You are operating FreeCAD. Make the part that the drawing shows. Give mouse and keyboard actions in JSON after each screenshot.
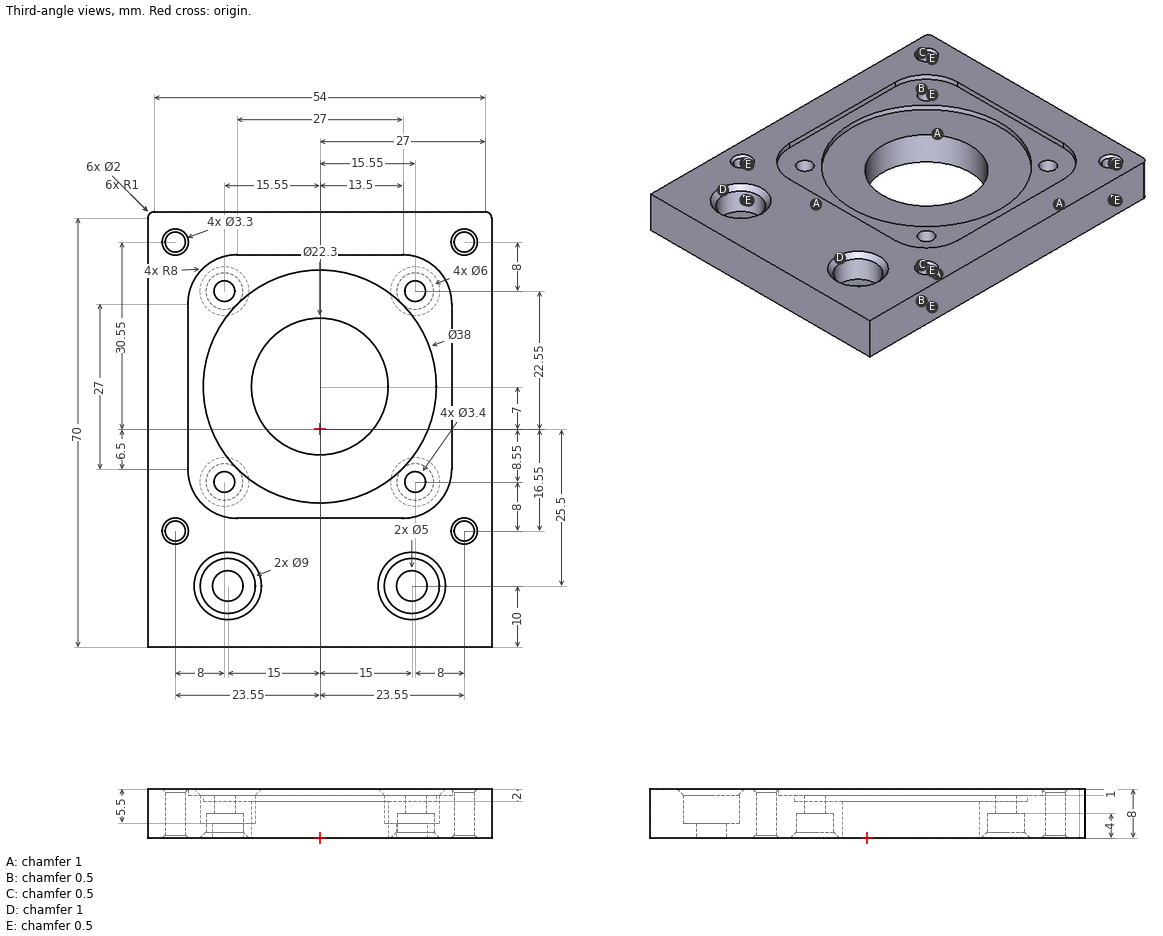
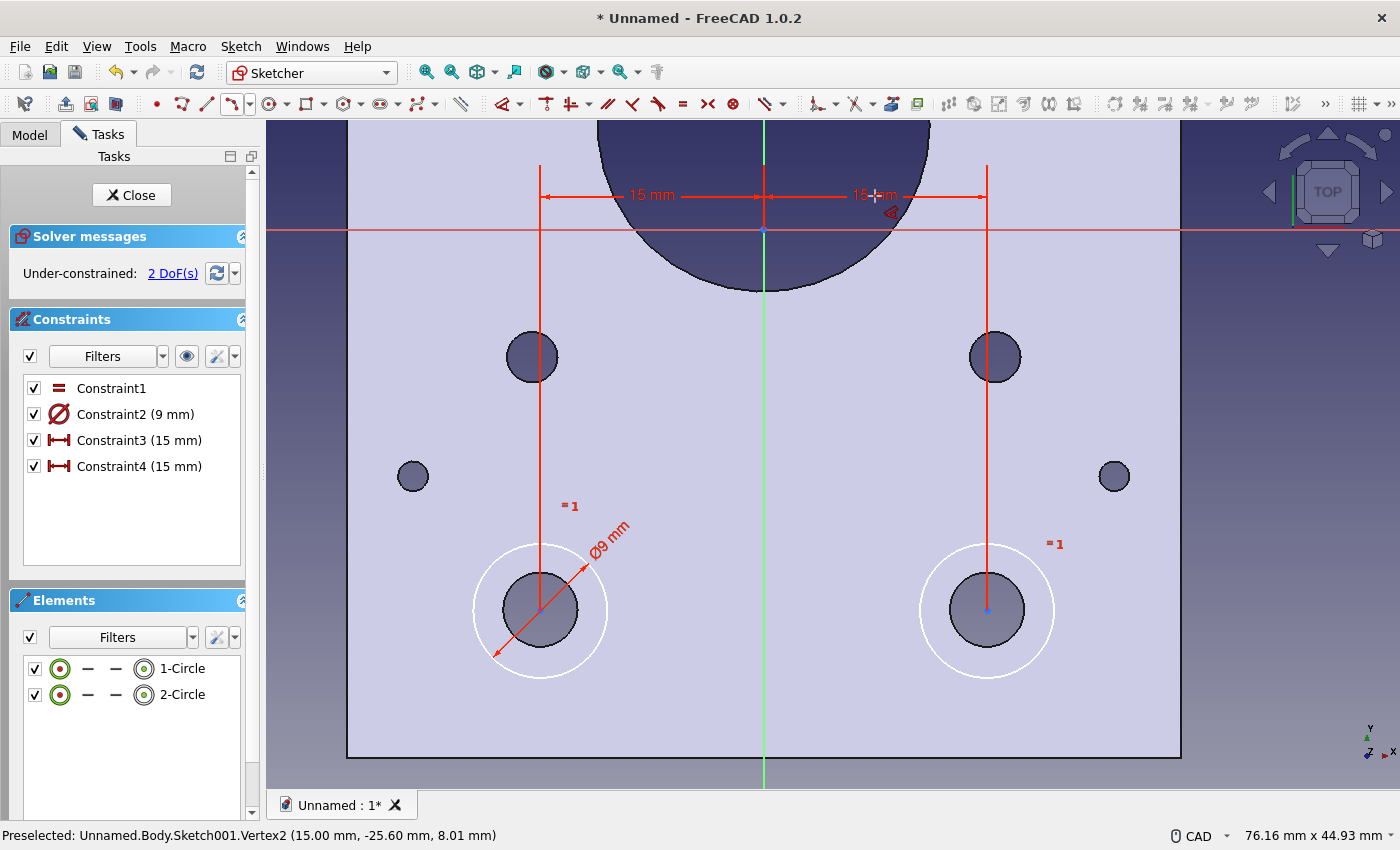
{"action": "left_click", "coordinate": [540, 611]}
{"action": "left_click", "coordinate": [506, 420]}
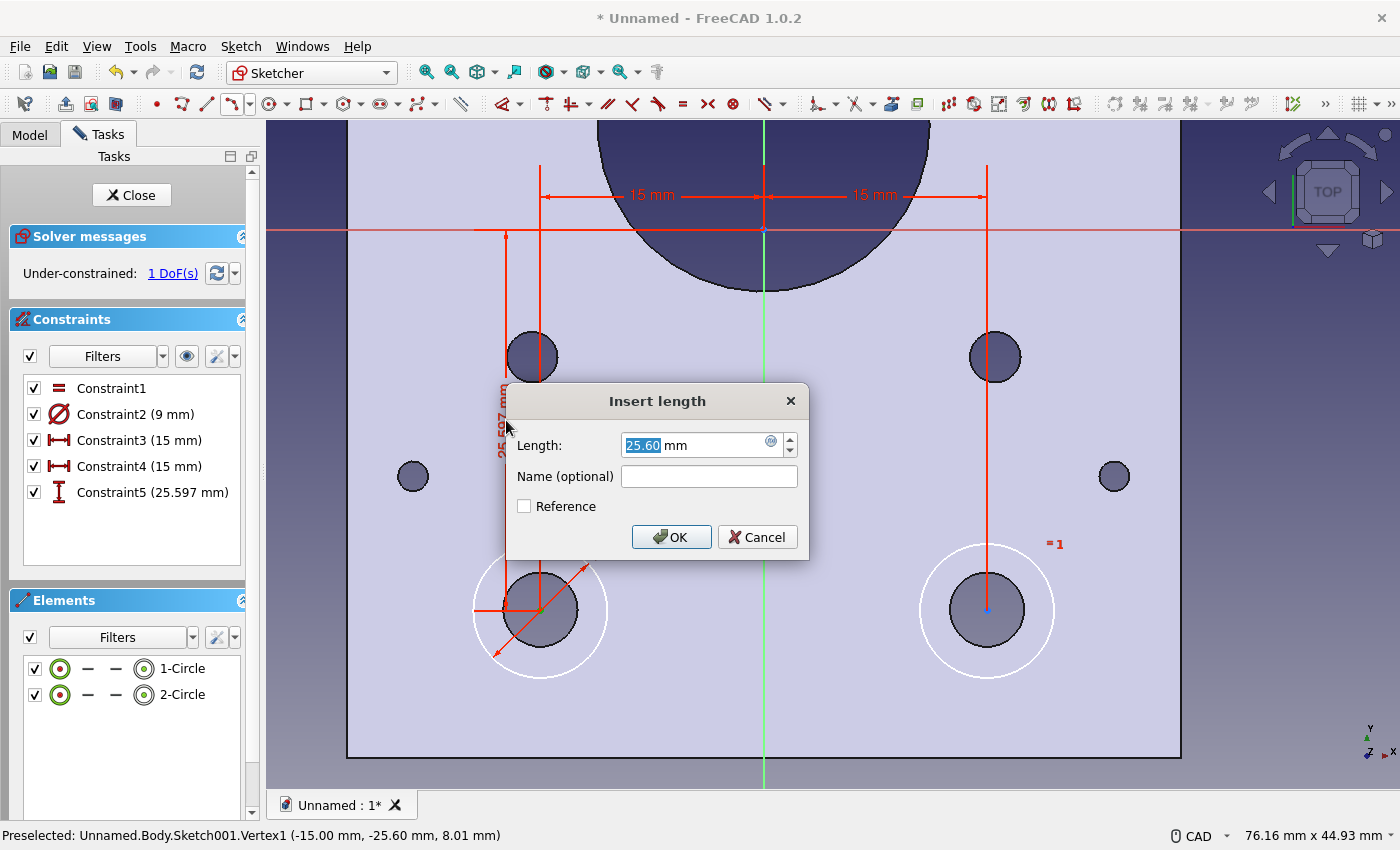
{"action": "type", "text": "25.5"}
{"action": "key", "text": "Return"}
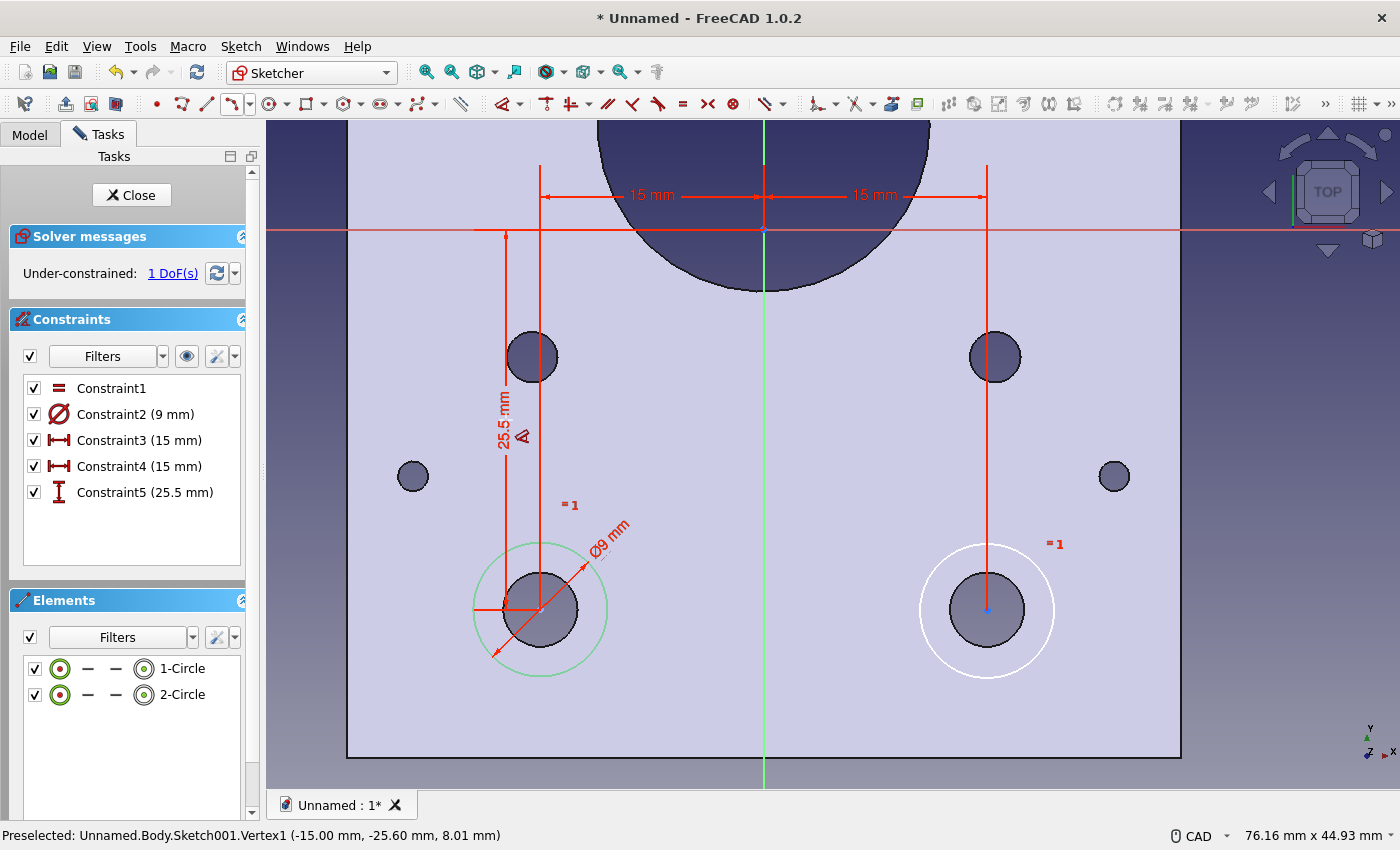
{"action": "left_click", "coordinate": [987, 611]}
{"action": "left_click", "coordinate": [1021, 420]}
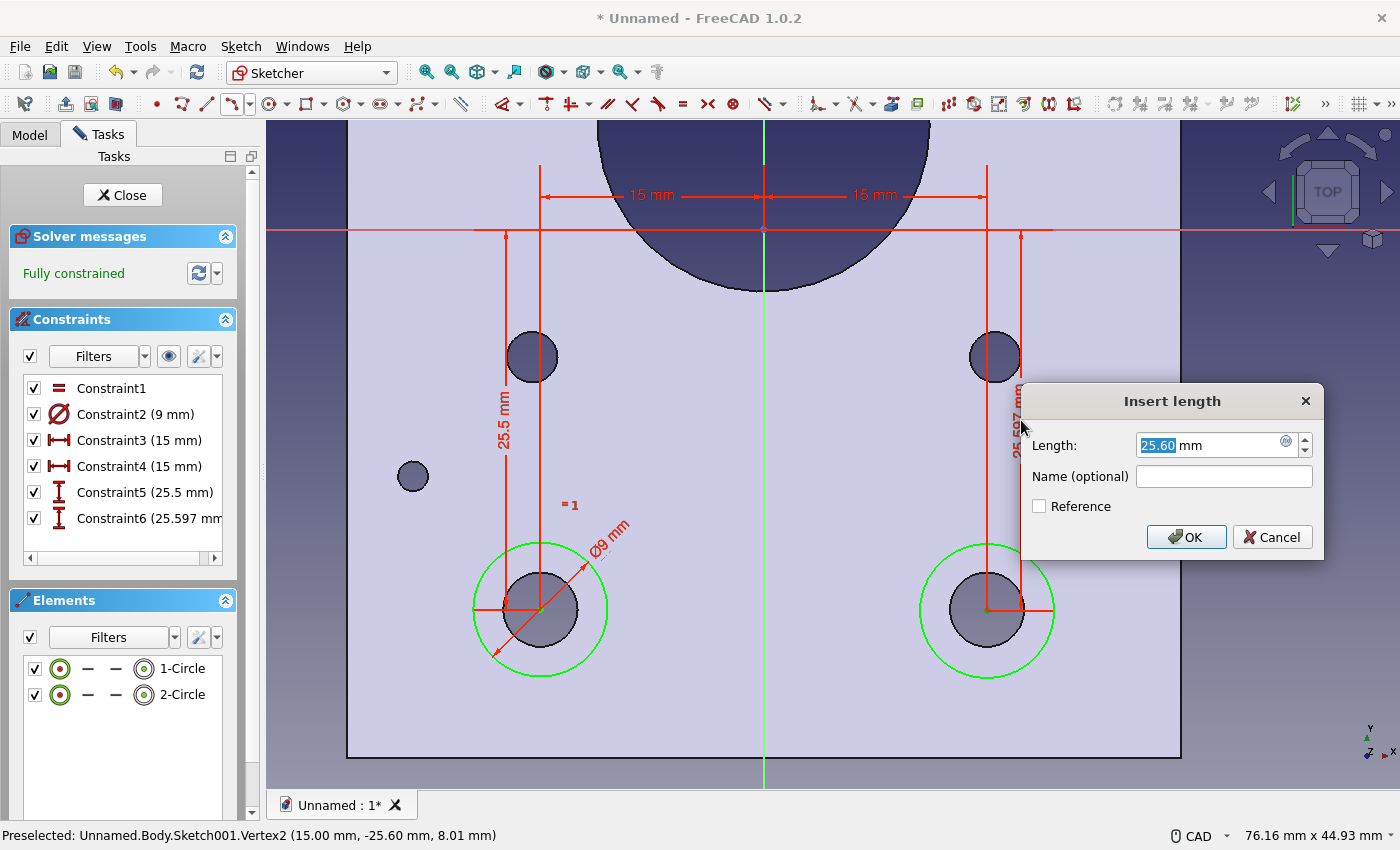
{"action": "type", "text": "25.5"}
{"action": "key", "text": "Return"}
{"action": "key", "text": "Escape"}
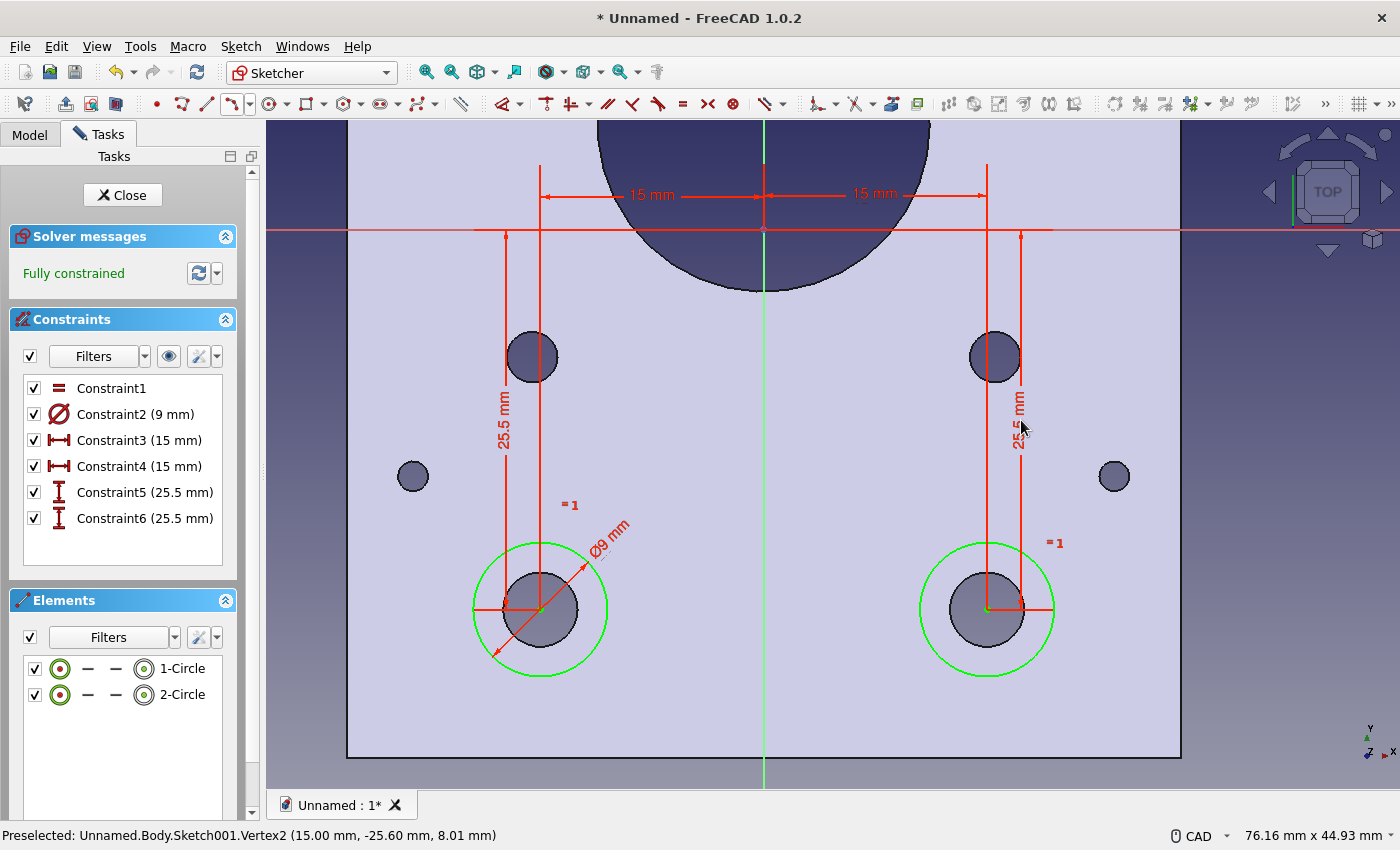
{"action": "left_click", "coordinate": [123, 195]}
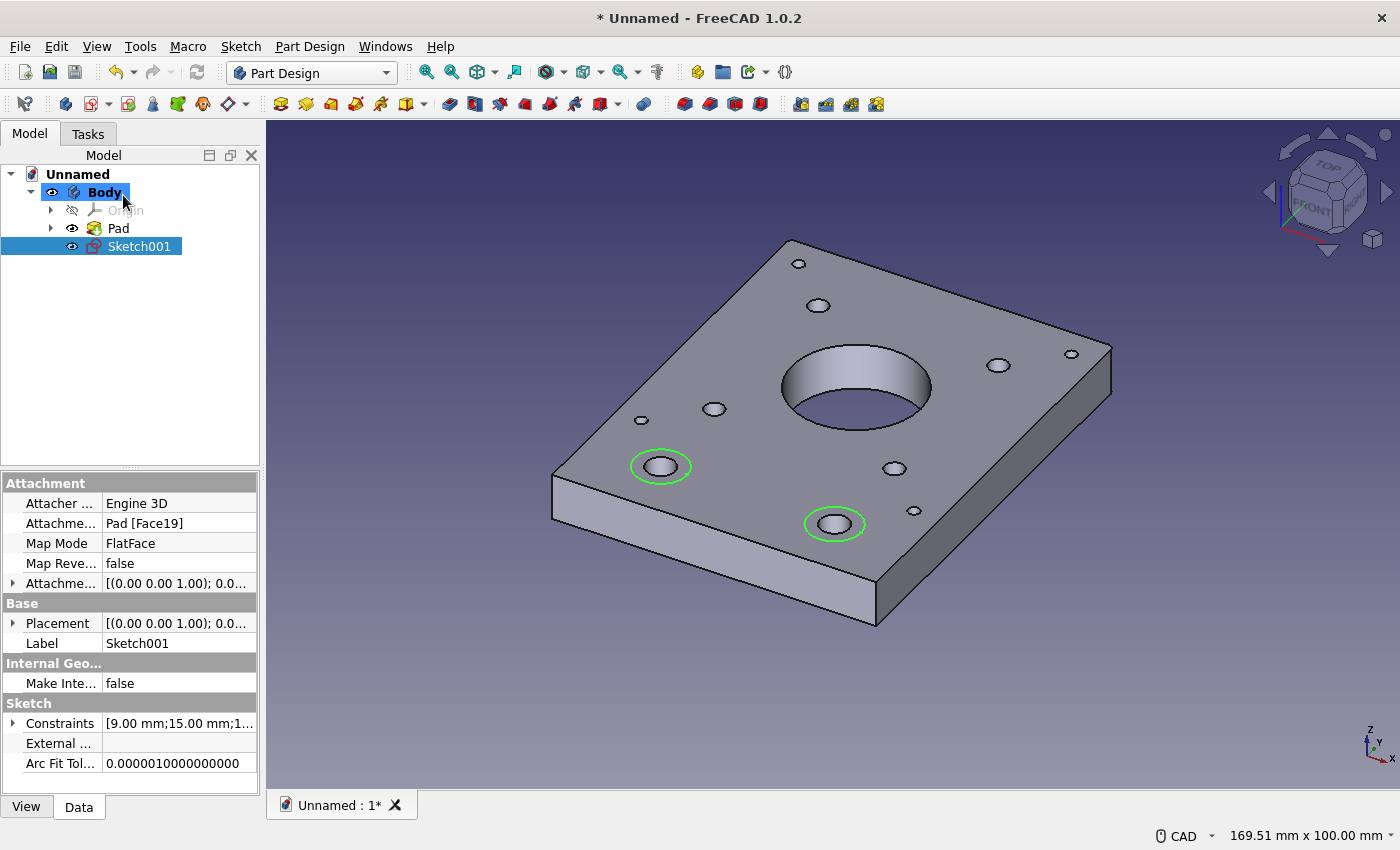
{"action": "left_click", "coordinate": [450, 104]}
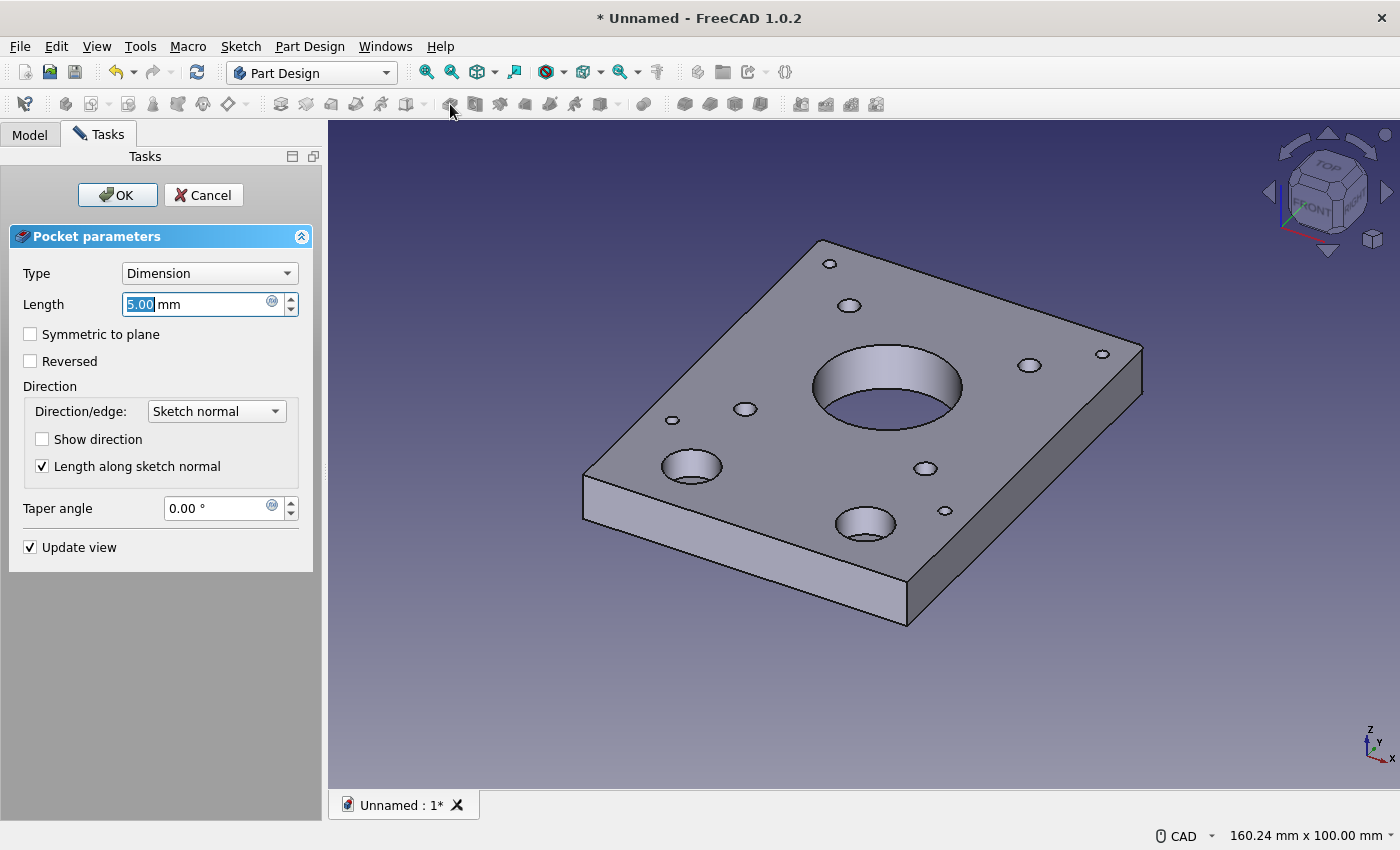
{"action": "type", "text": "5.5"}
{"action": "key", "text": "Tab"}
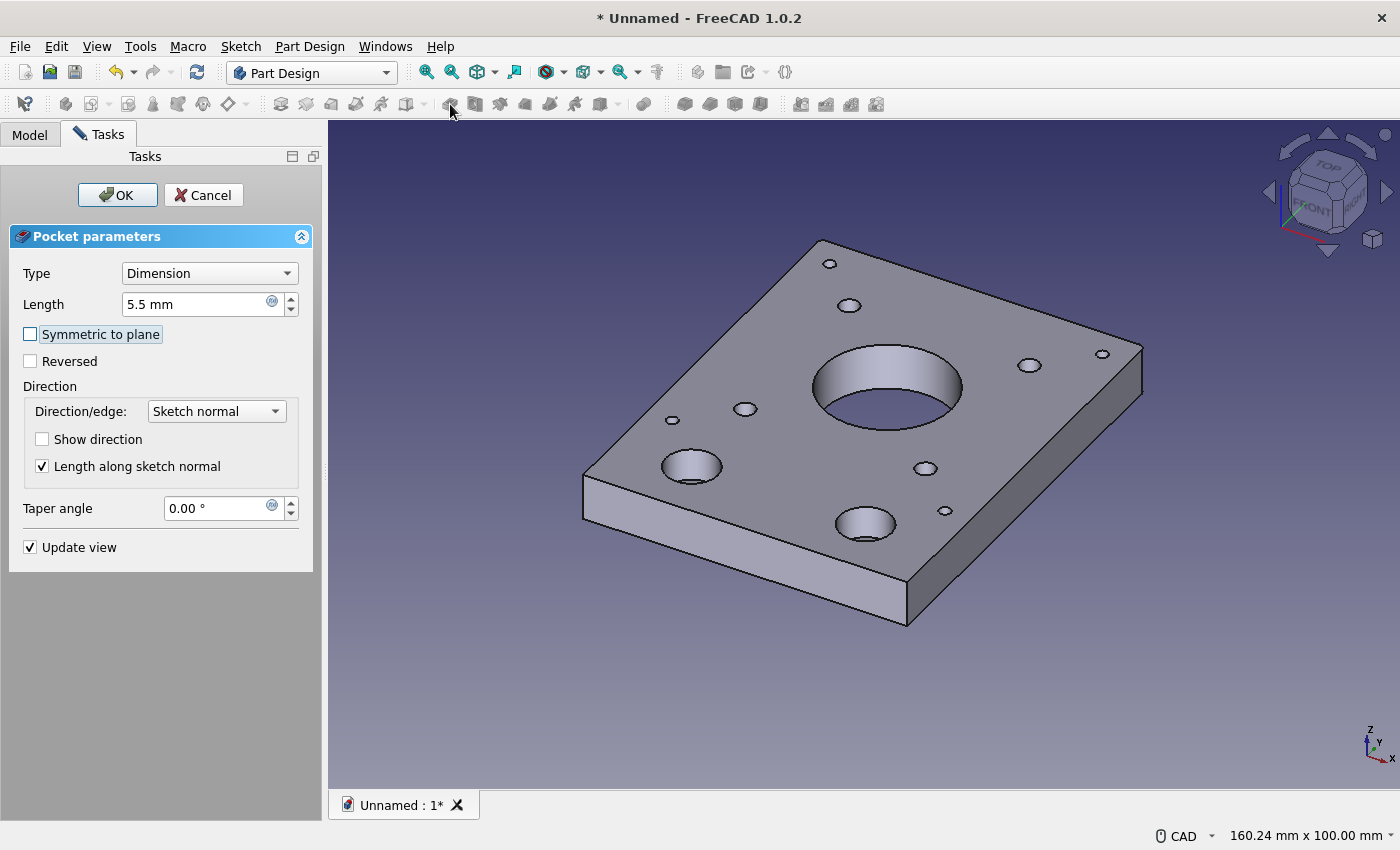
{"action": "left_click", "coordinate": [118, 195]}